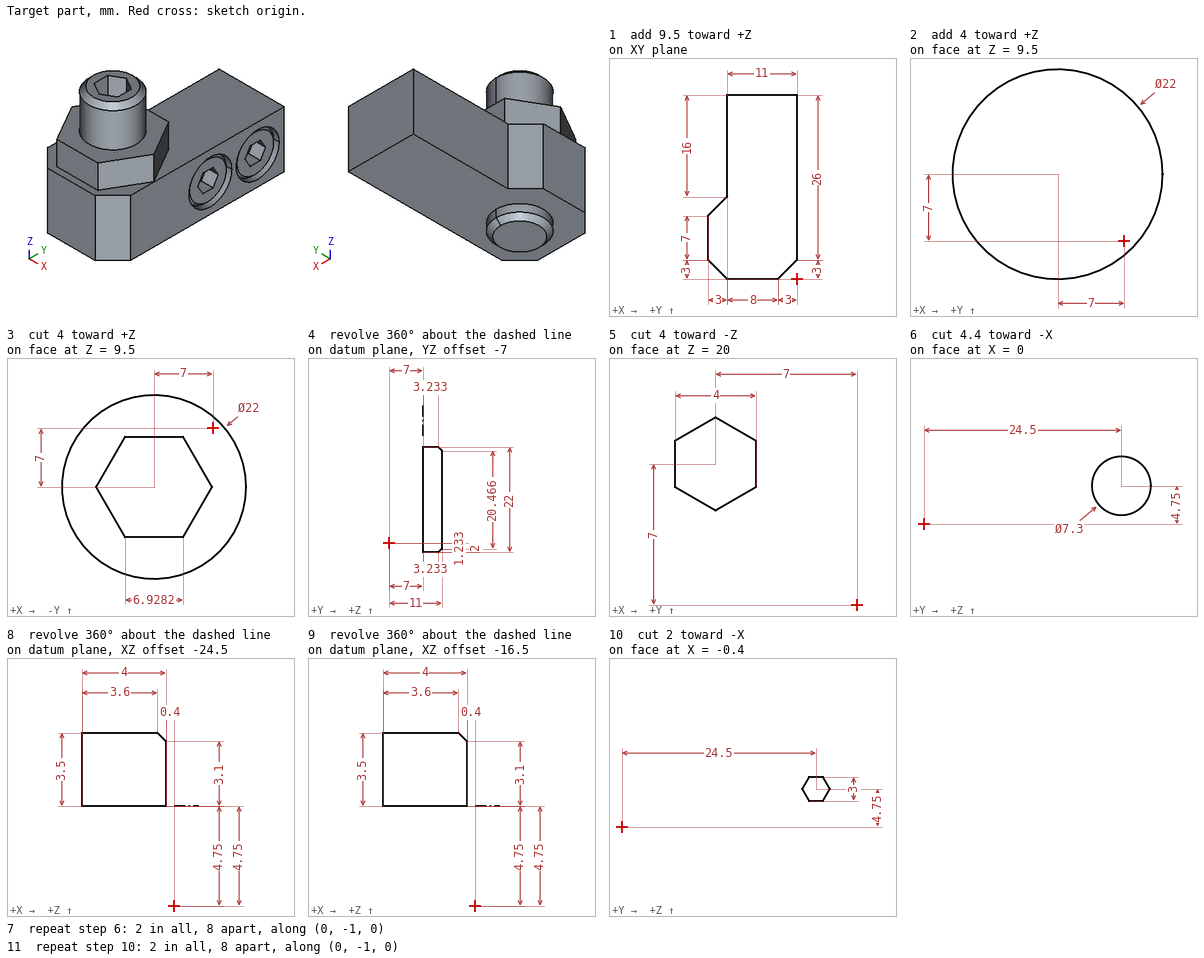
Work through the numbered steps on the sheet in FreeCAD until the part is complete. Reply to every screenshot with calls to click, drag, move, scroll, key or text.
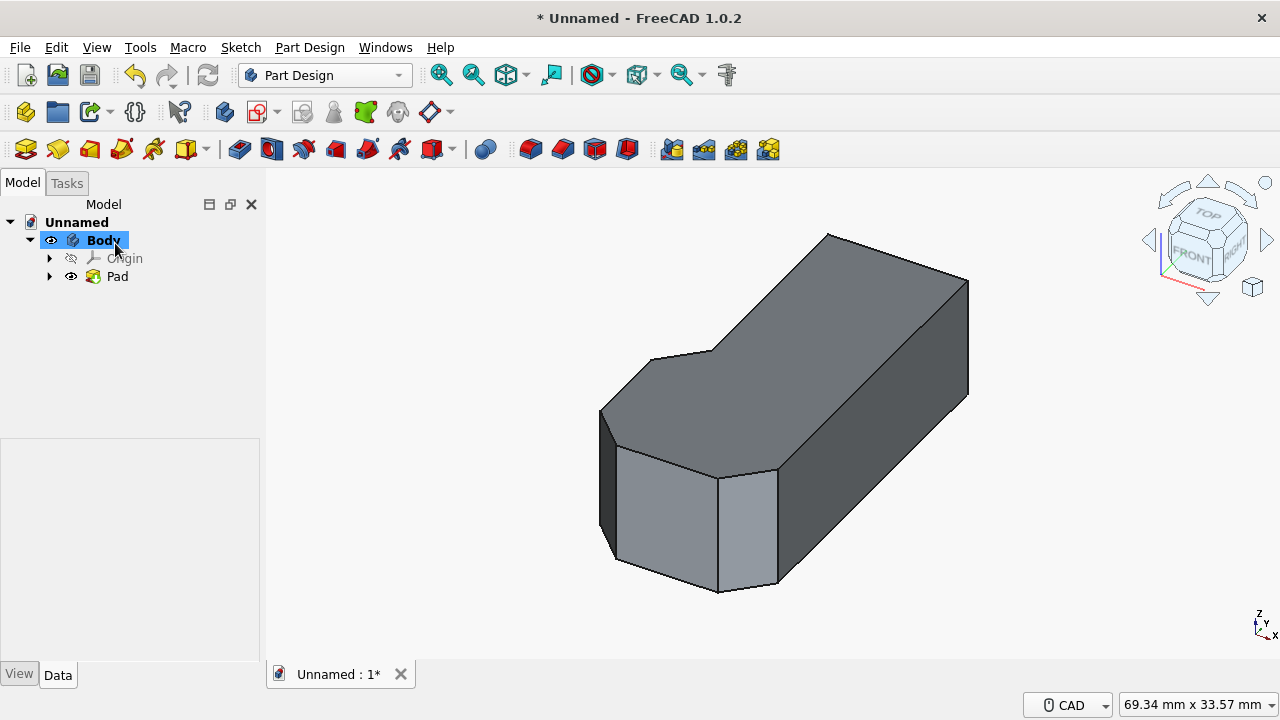
click(712, 416)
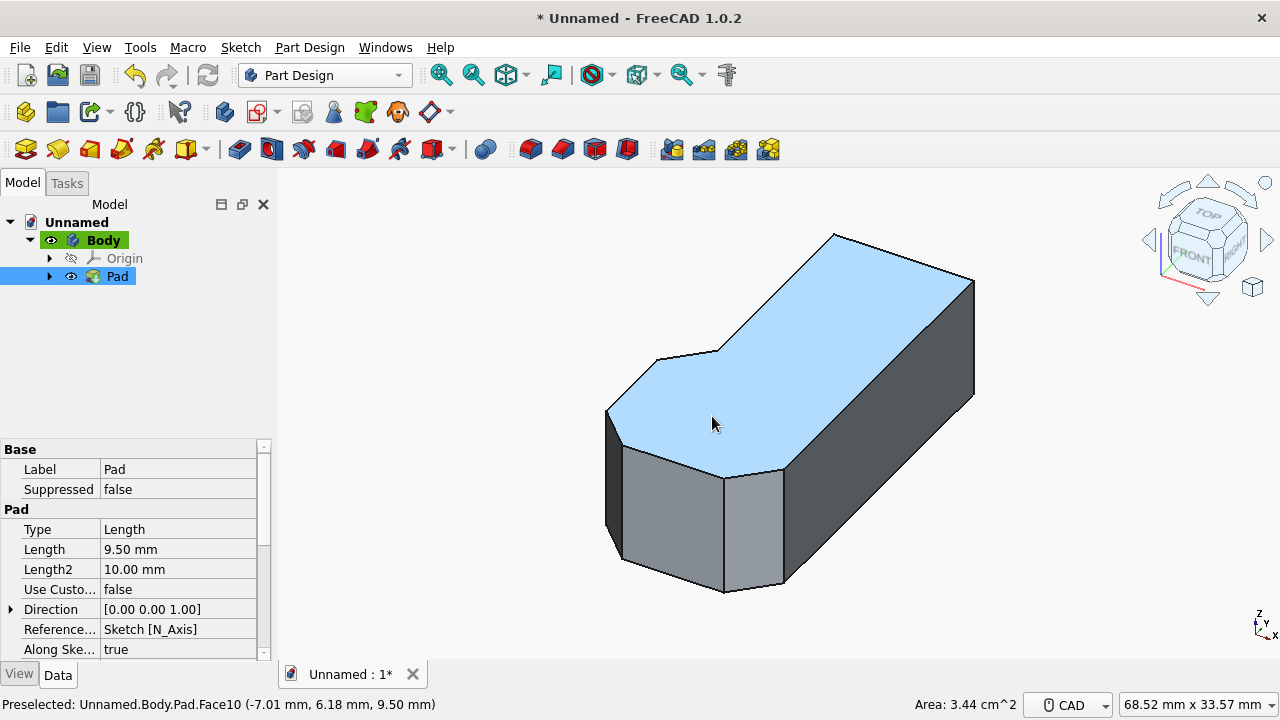
click(258, 112)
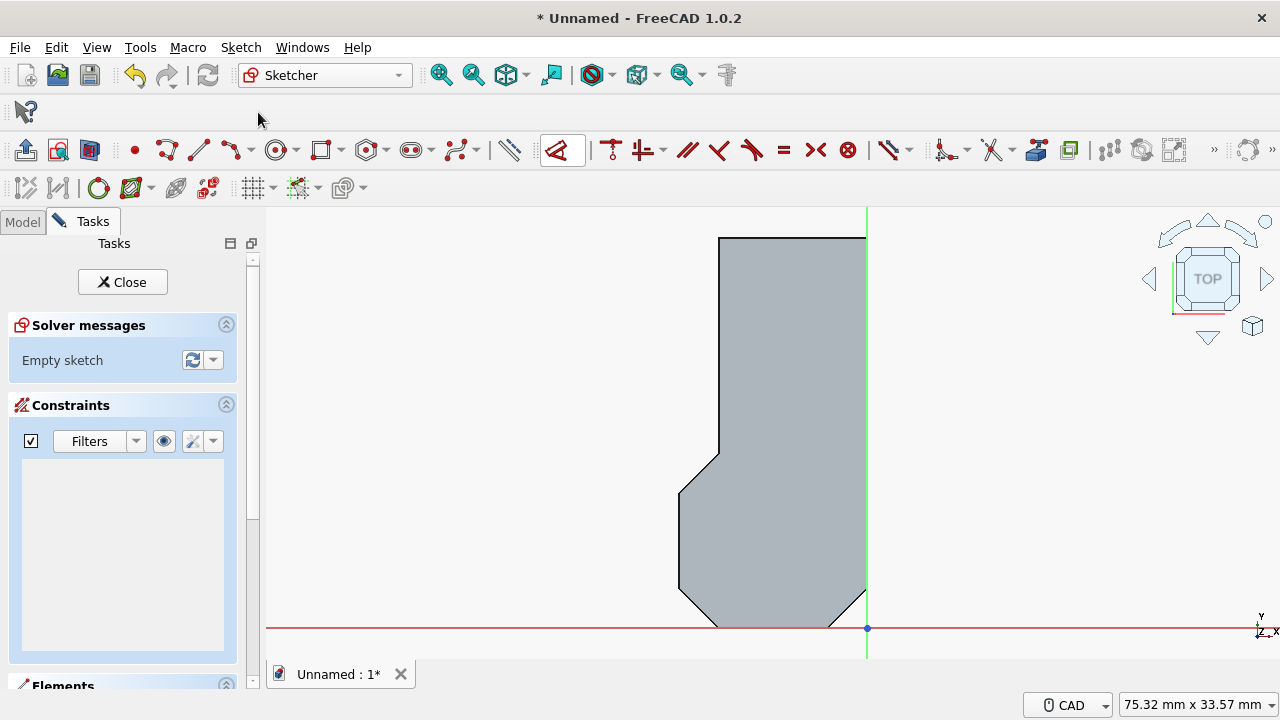
scroll(395, 235, down, 1)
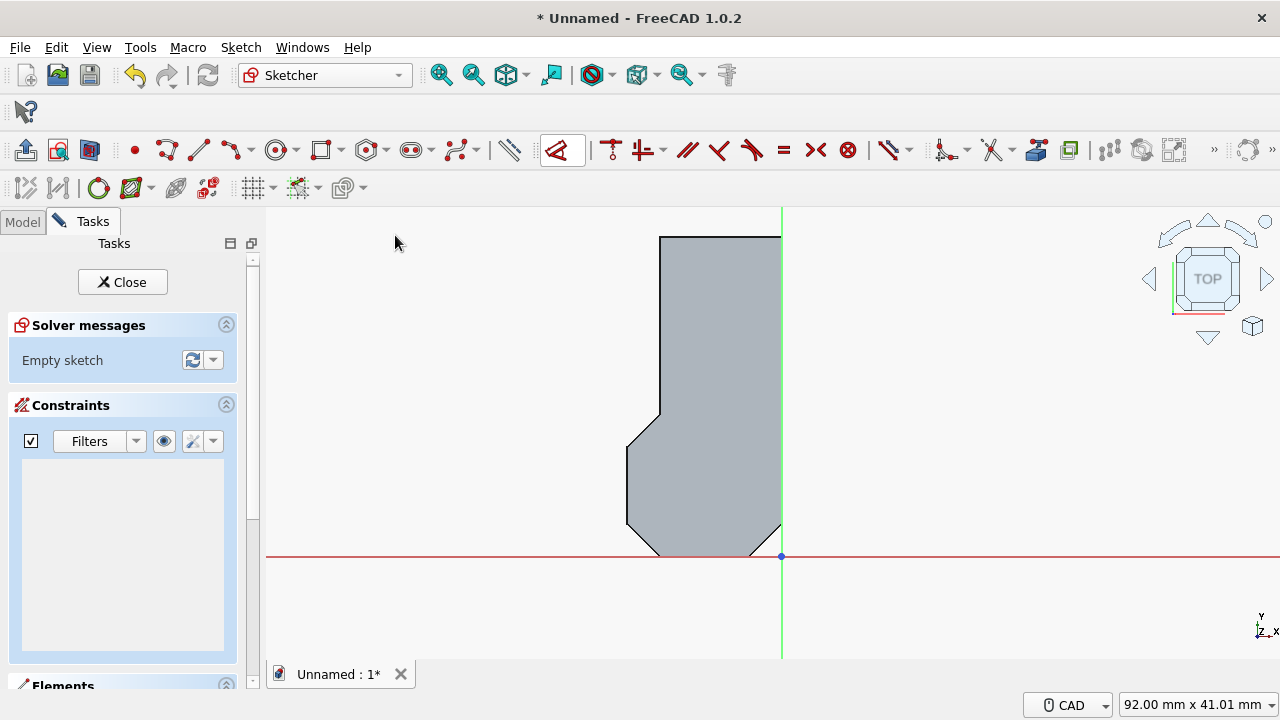
click(276, 150)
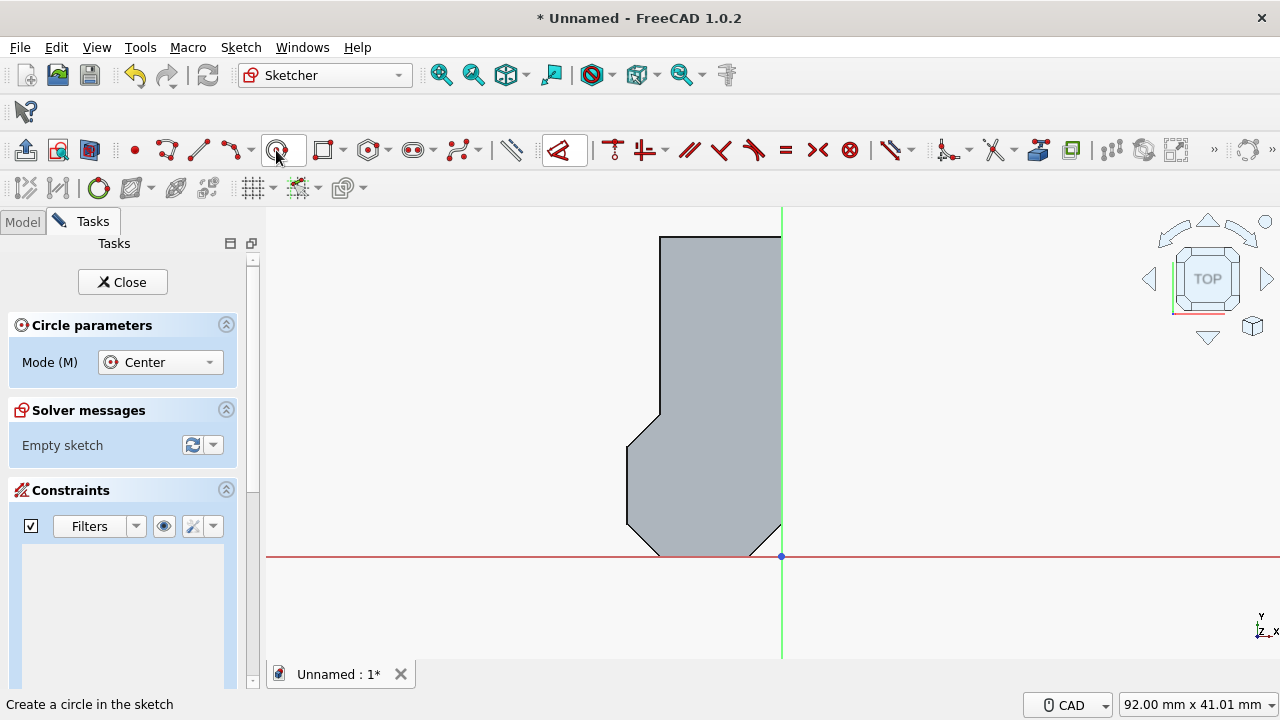
click(705, 480)
click(619, 394)
key(Escape)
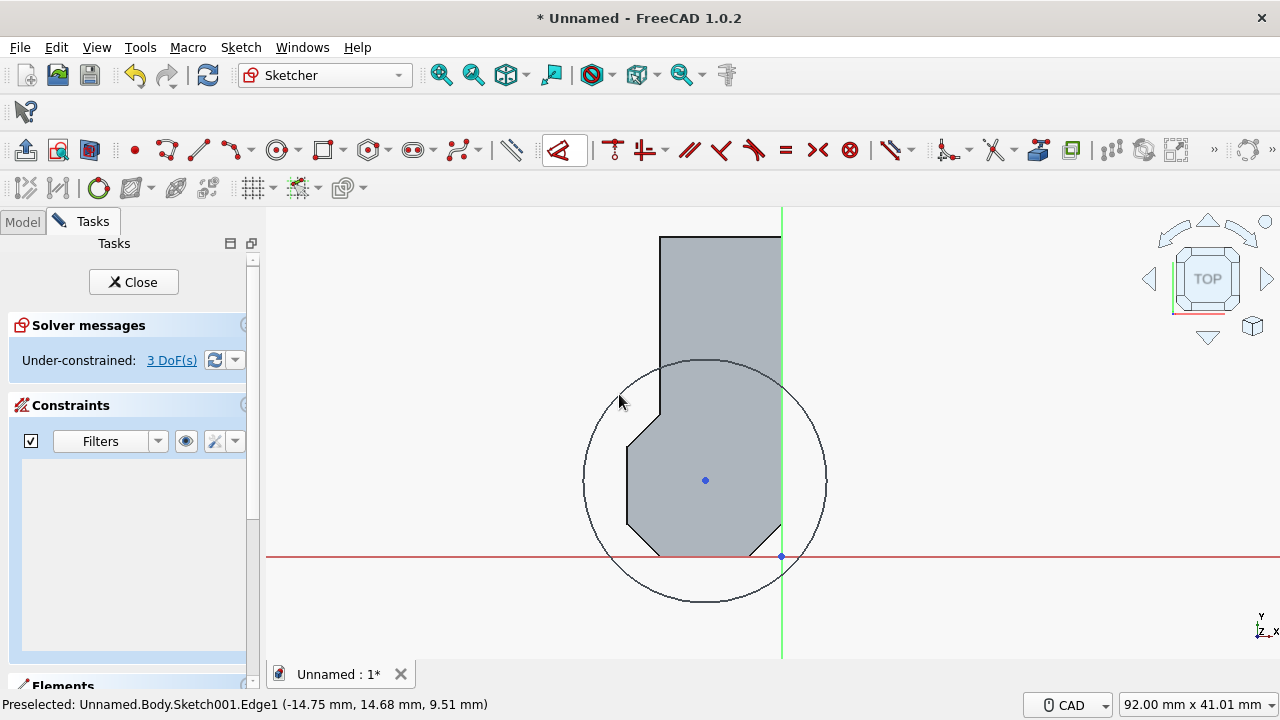
scroll(791, 395, up, 3)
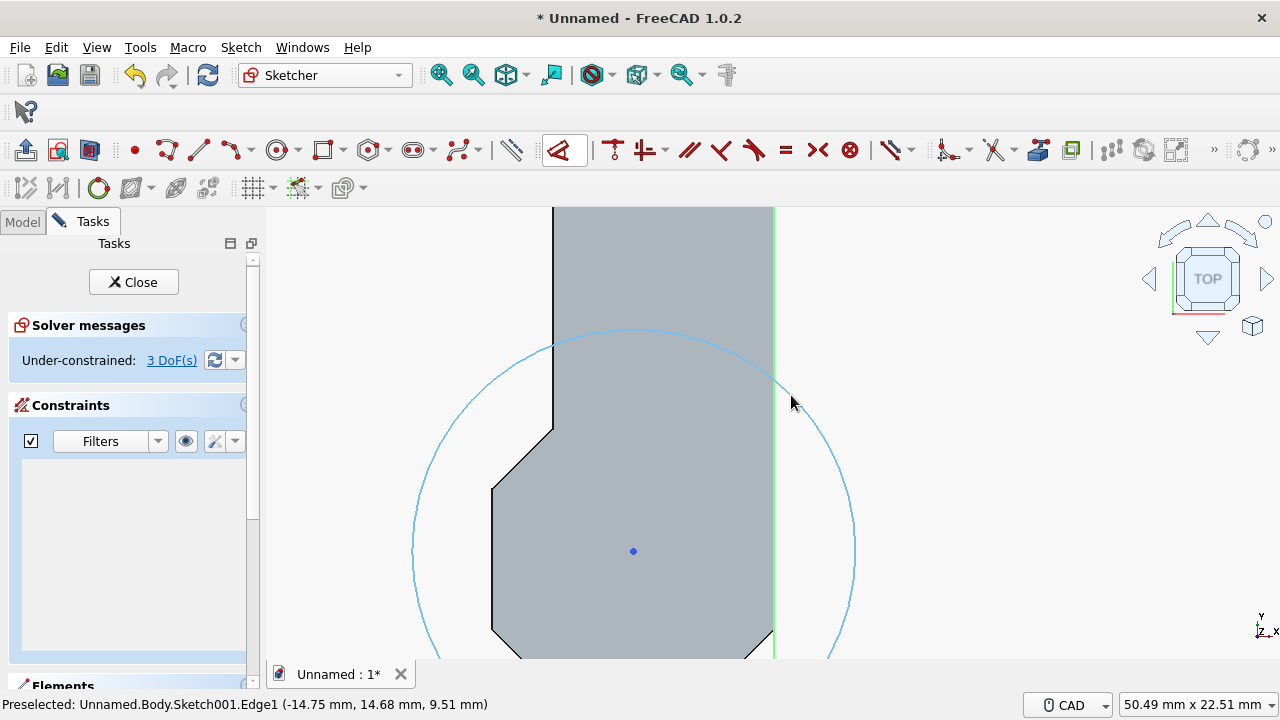
click(790, 394)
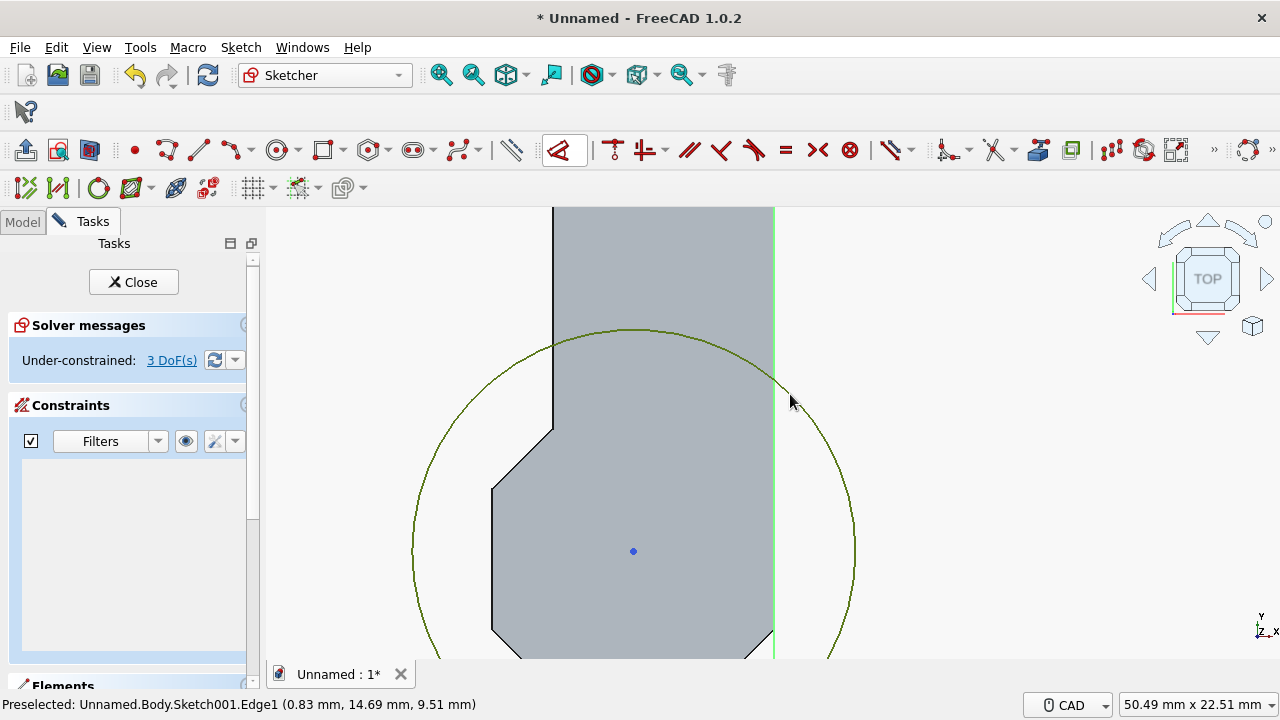
key(k)
key(o)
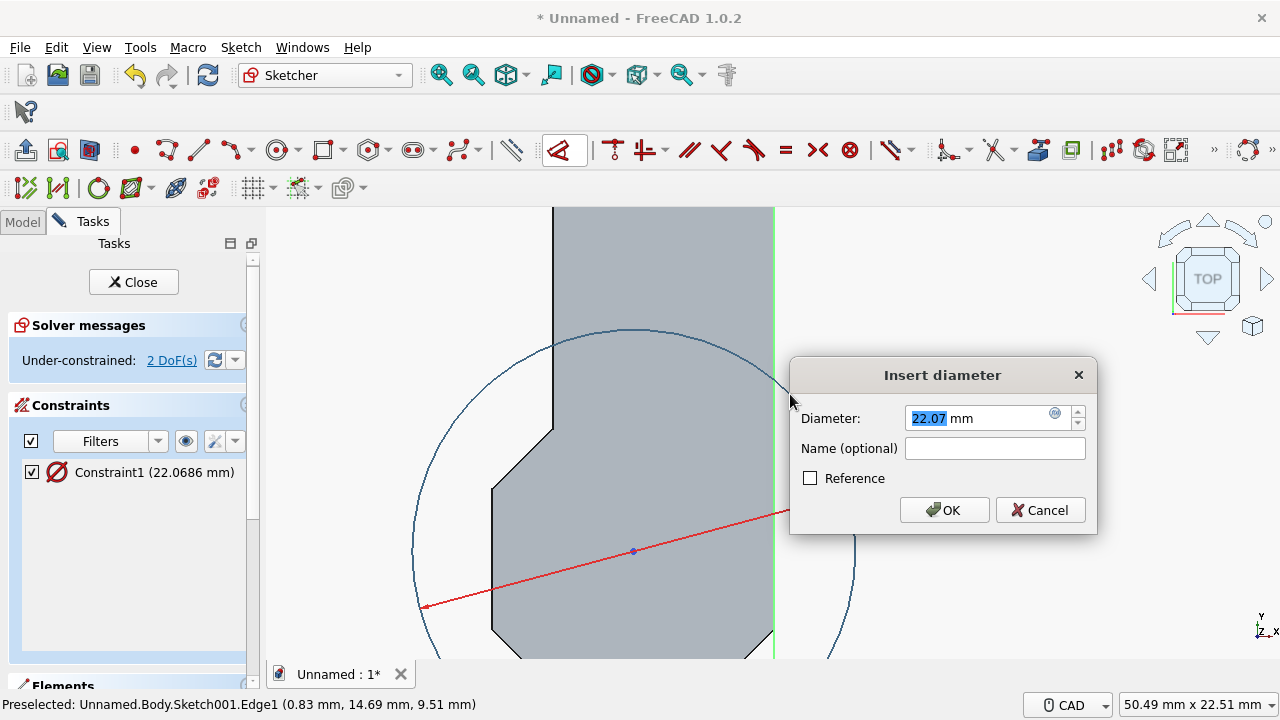
text(22)
key(Return)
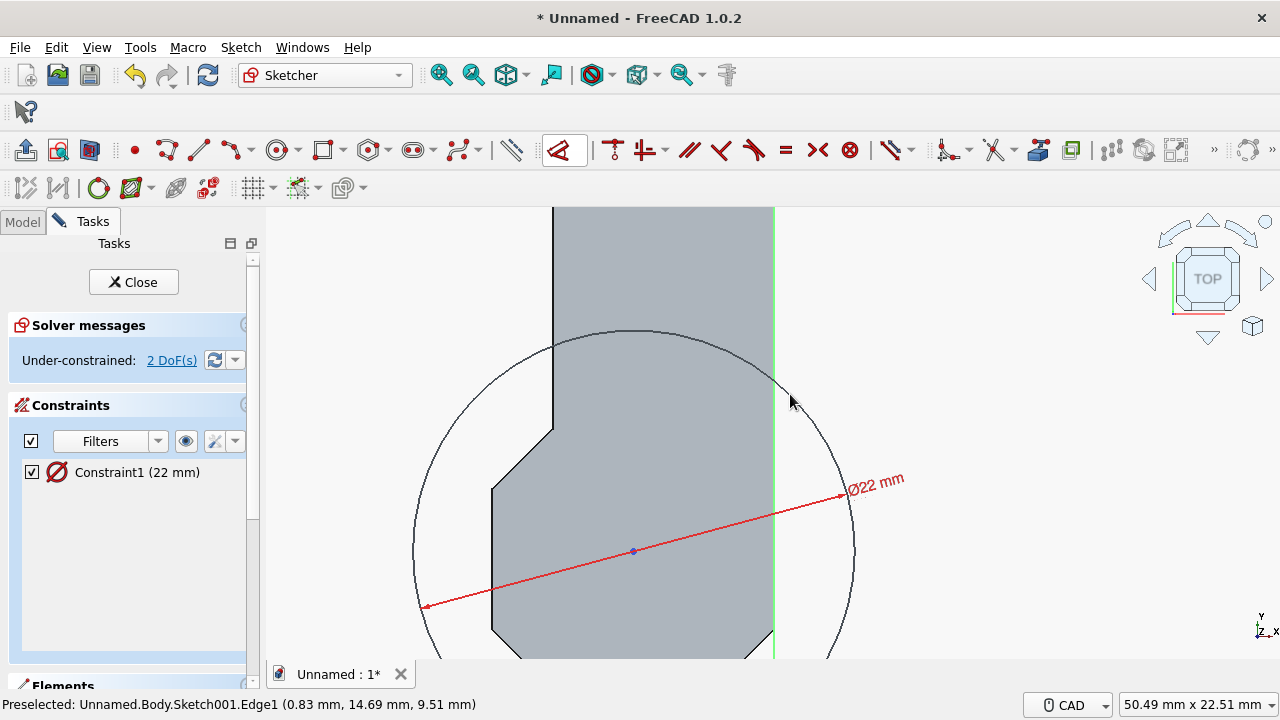
click(634, 551)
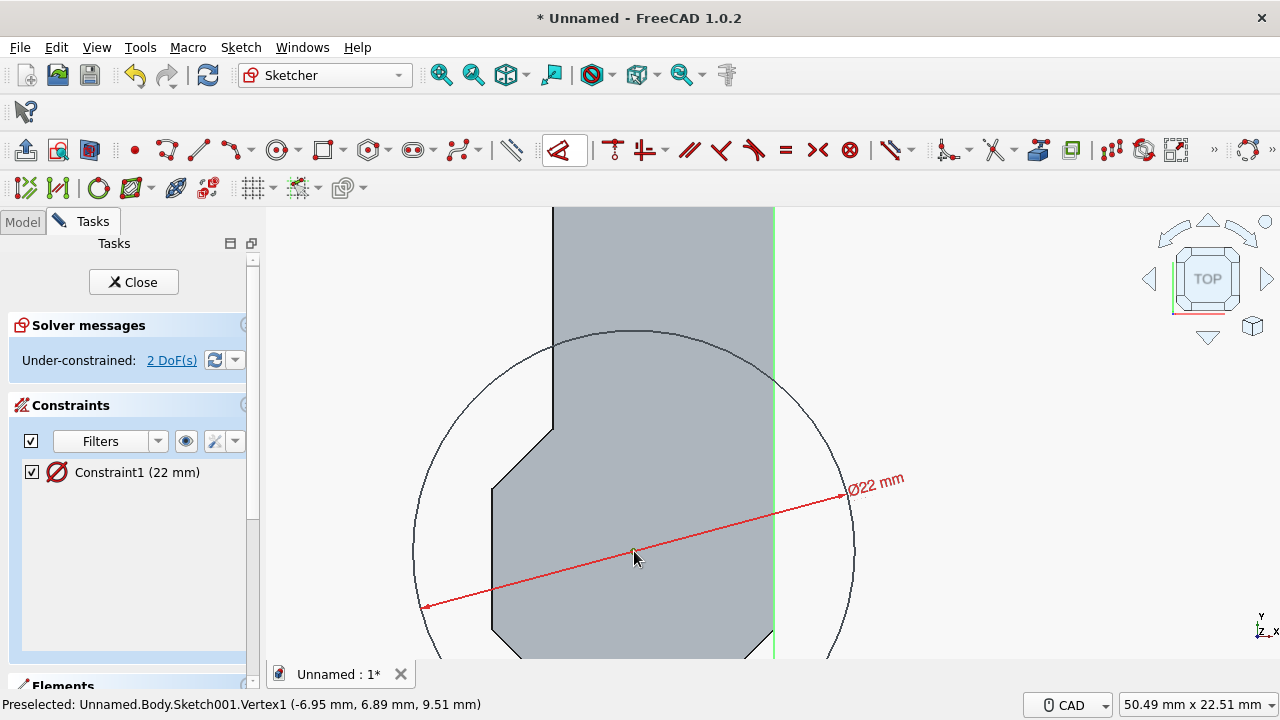
key(l)